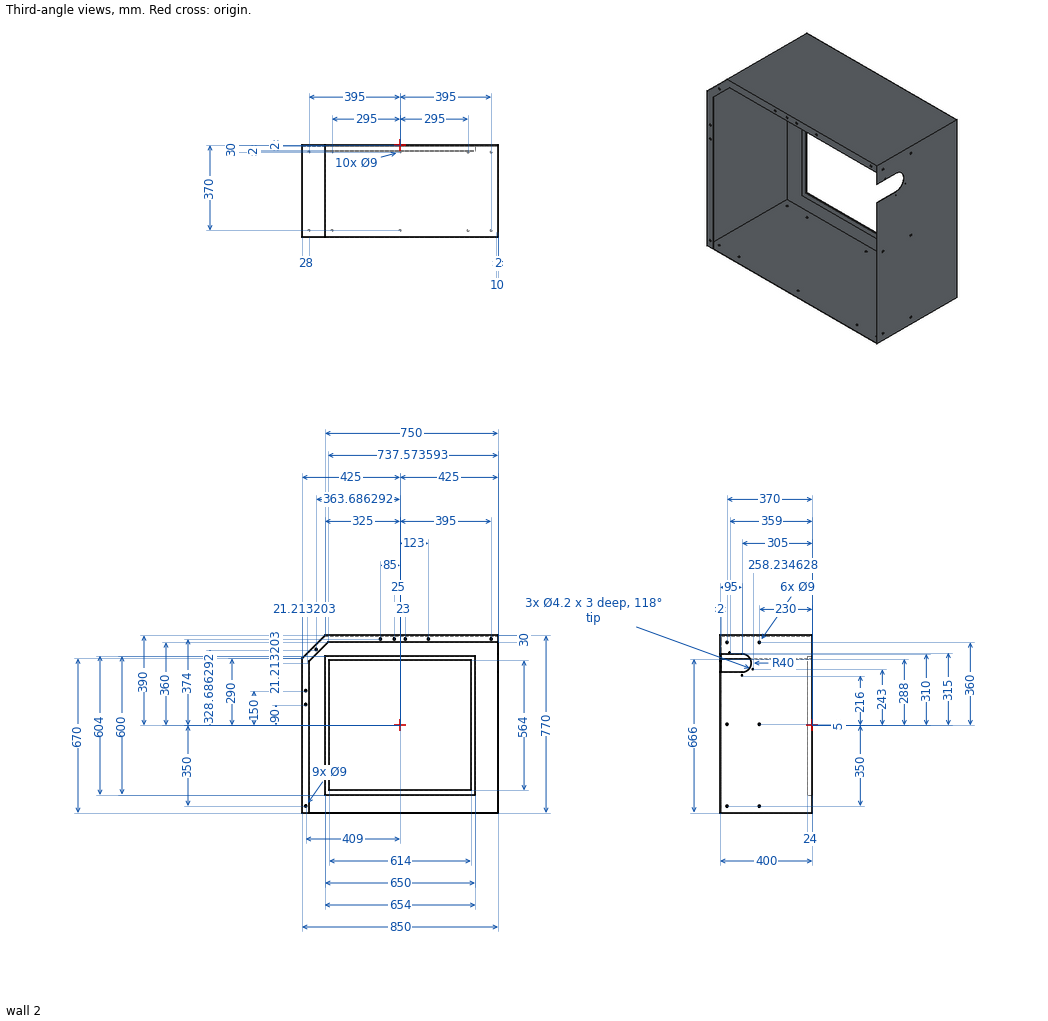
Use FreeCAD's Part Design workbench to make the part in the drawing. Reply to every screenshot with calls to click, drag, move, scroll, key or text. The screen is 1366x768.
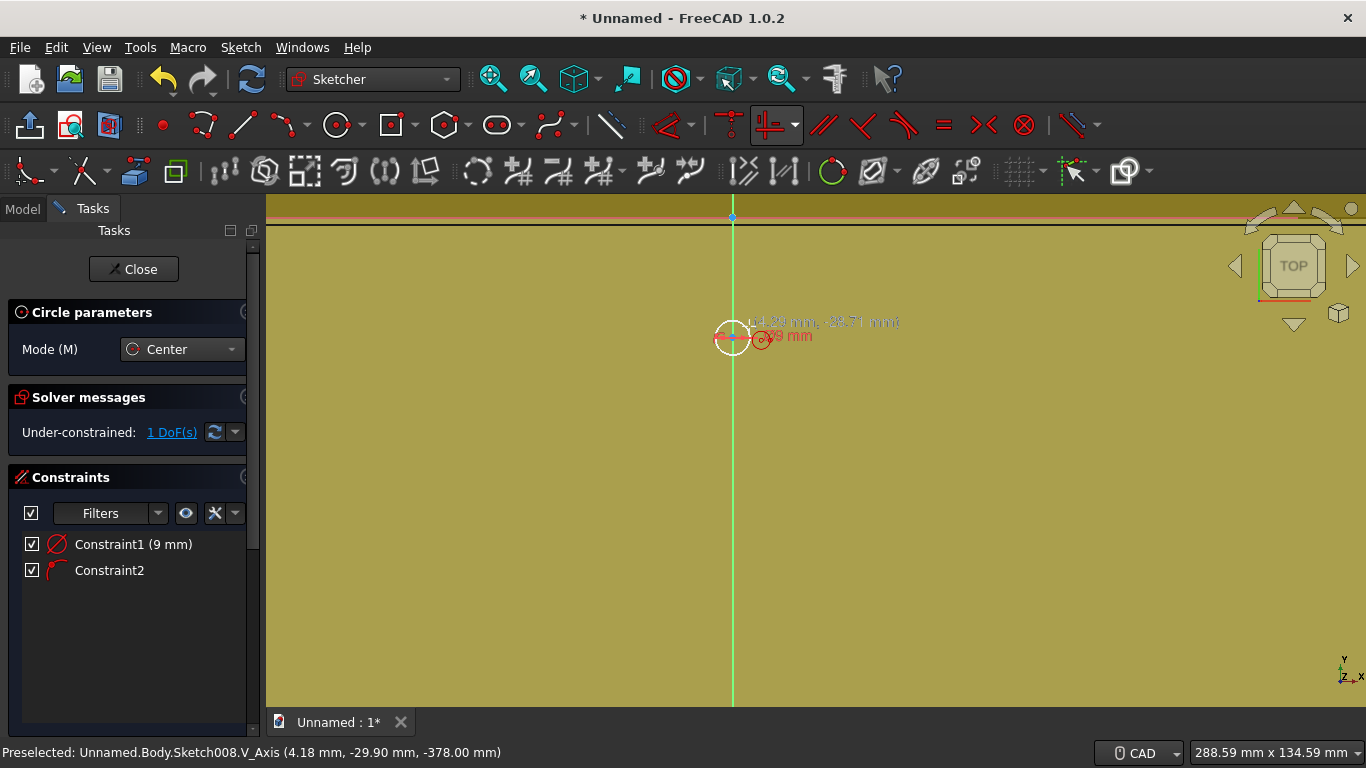
scroll(751, 329, down, 8)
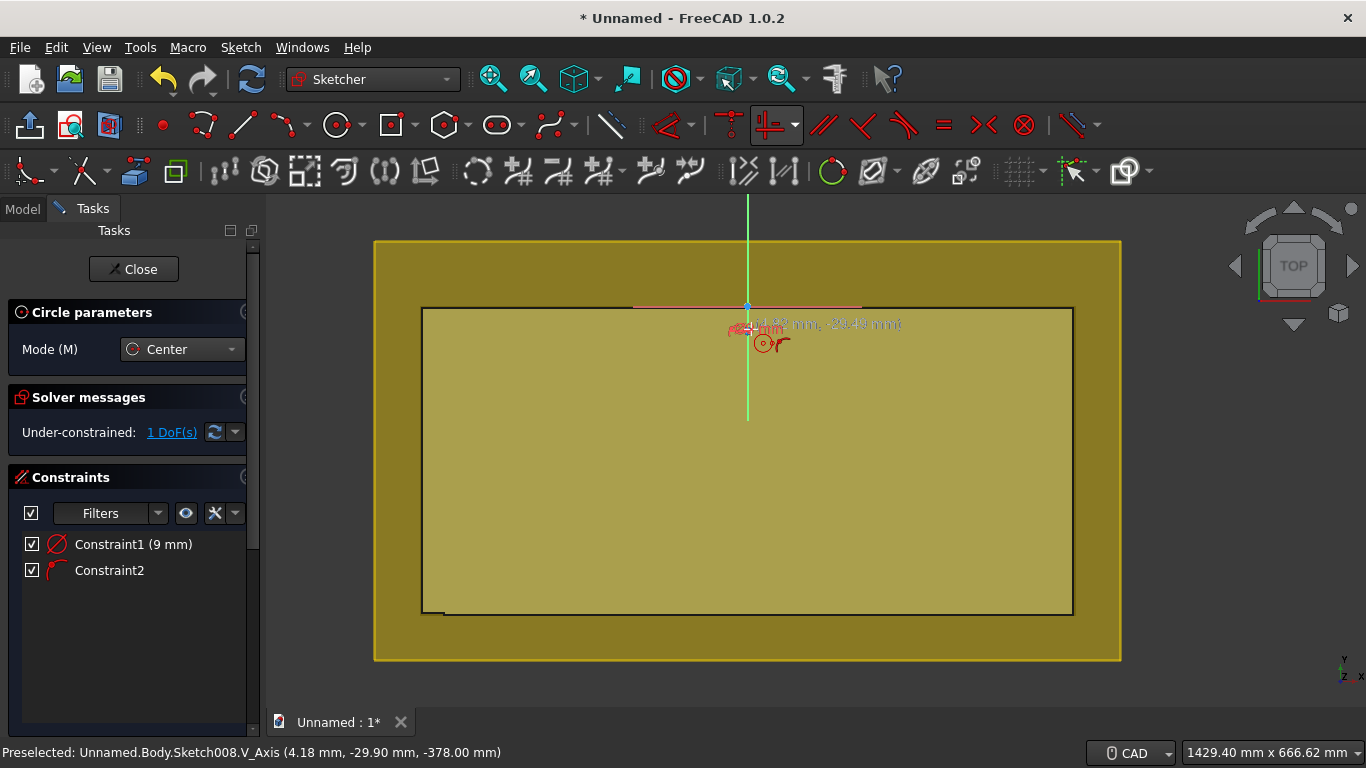
scroll(521, 330, up, 10)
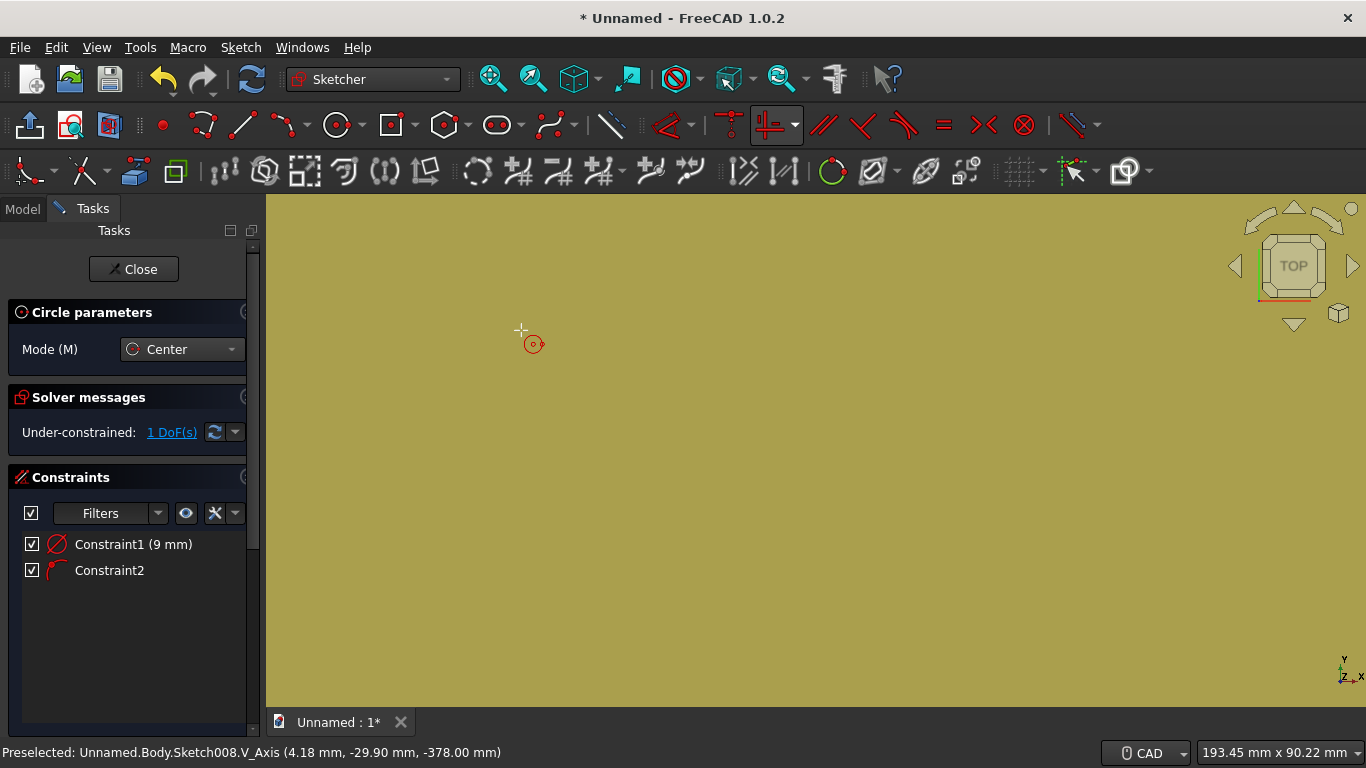
scroll(521, 330, down, 10)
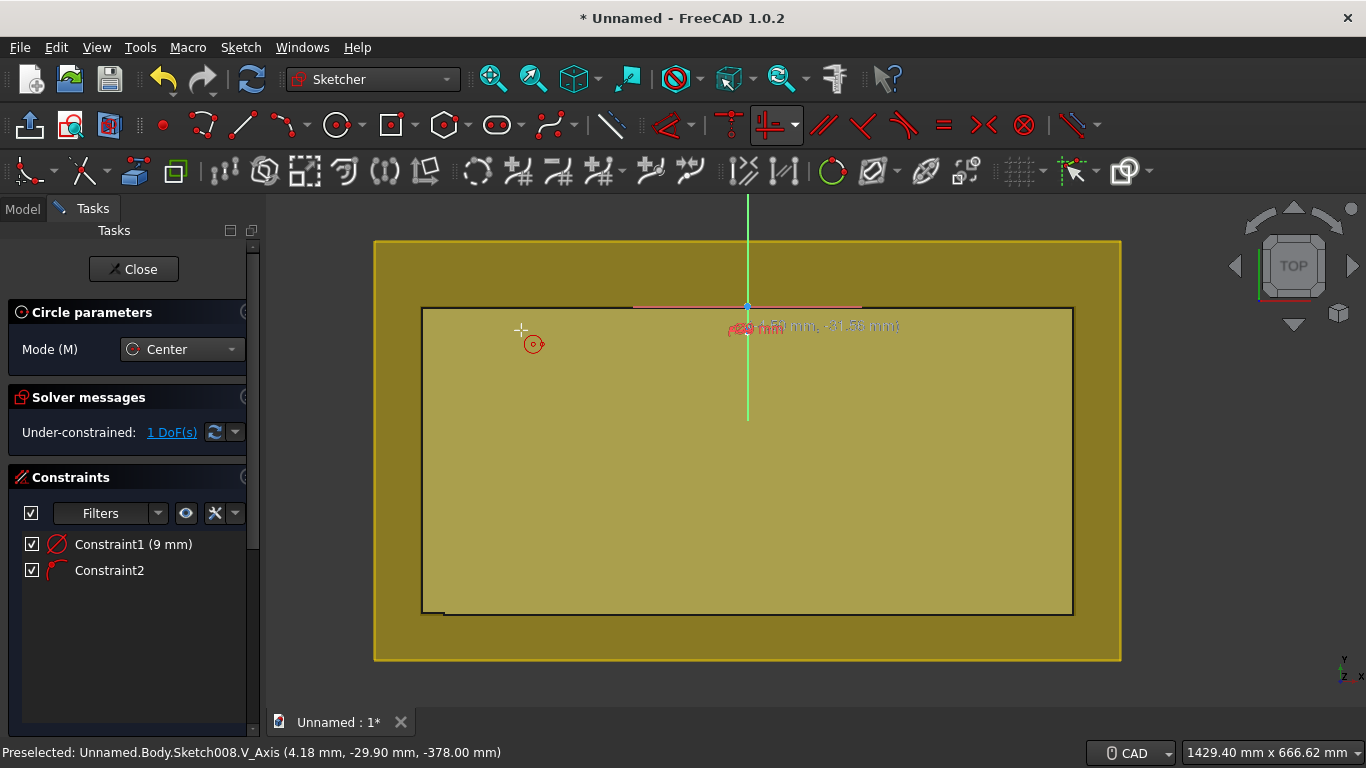
click(521, 330)
move(523, 327)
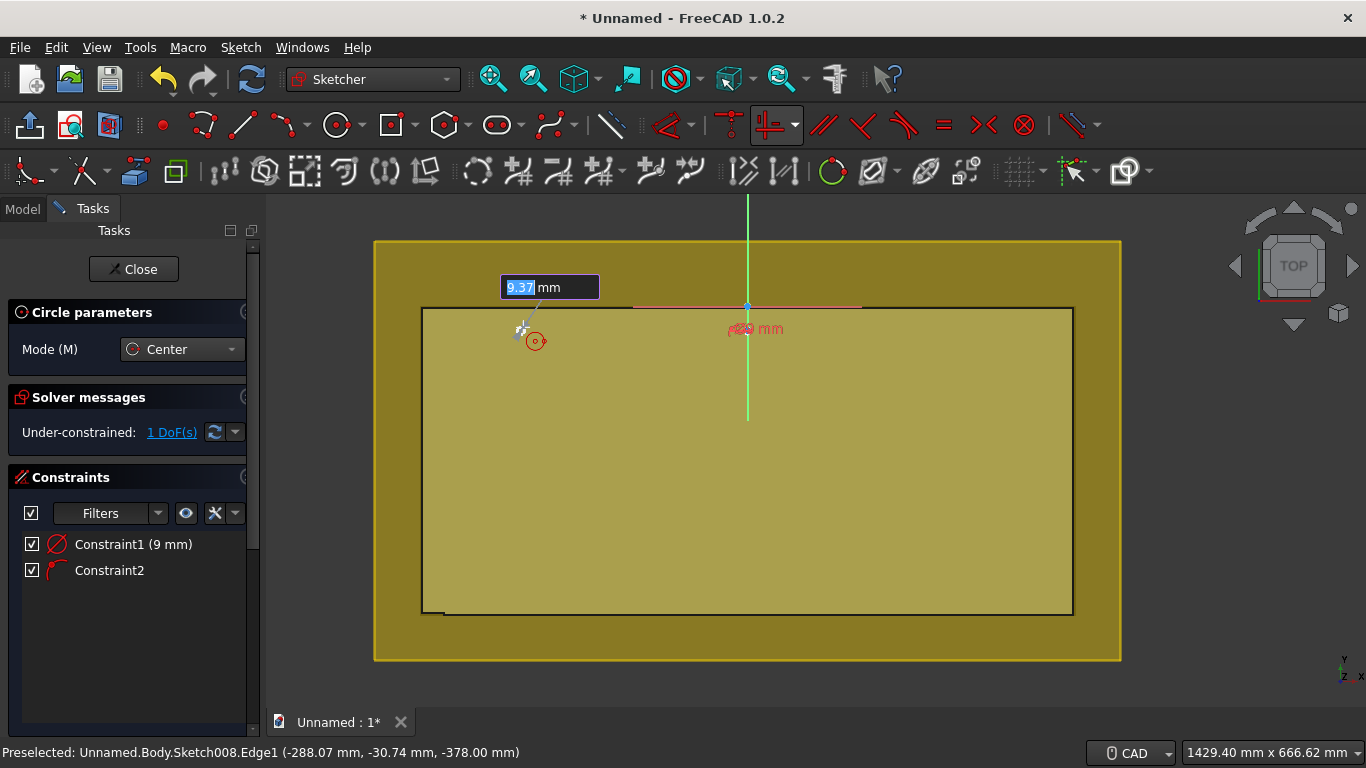
text(9)
key(Return)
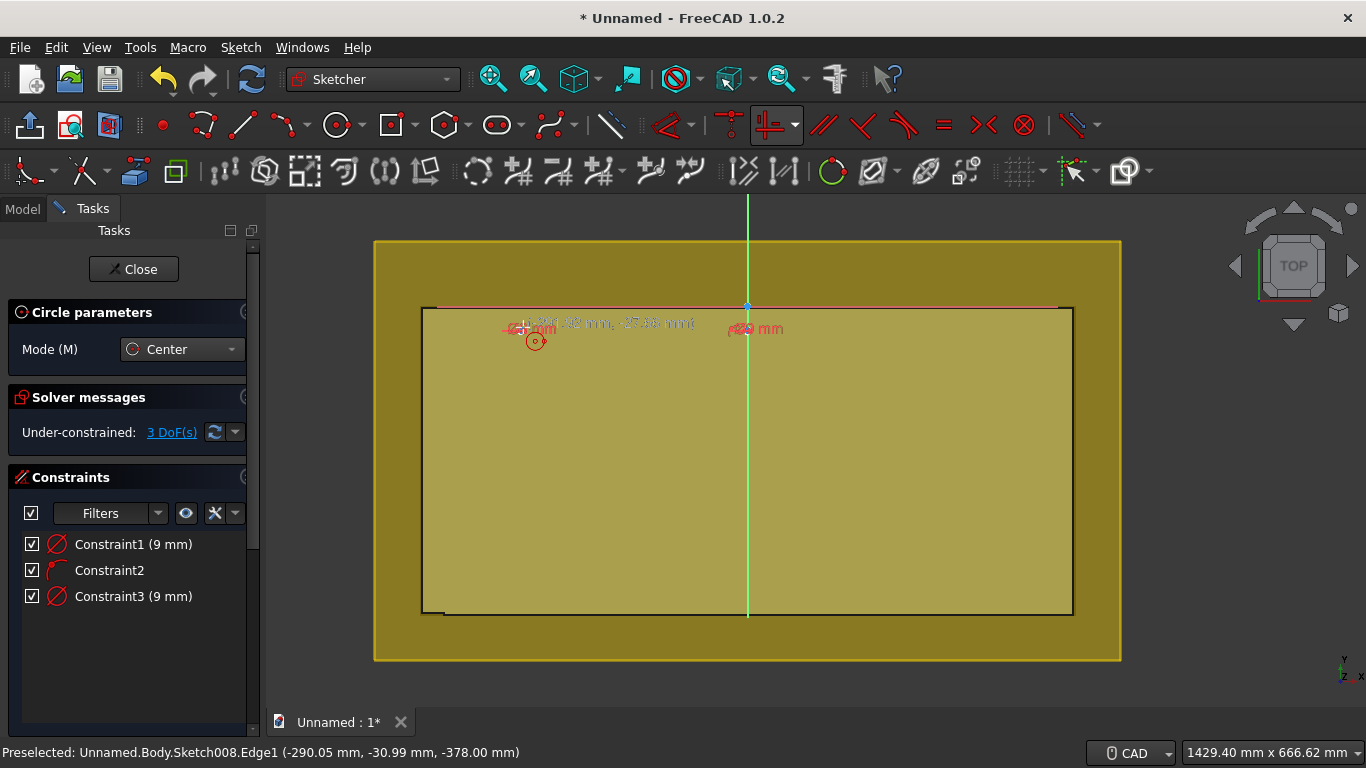
scroll(748, 591, up, 10)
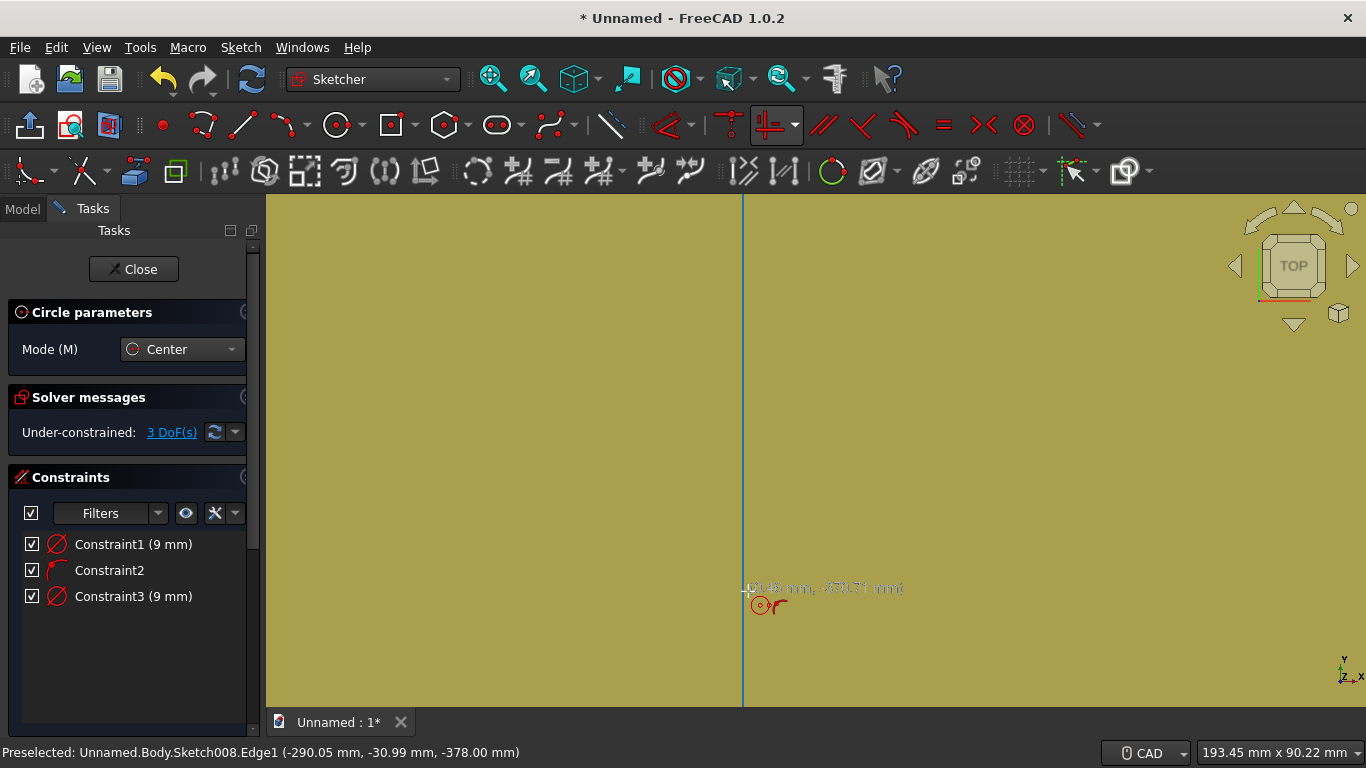
scroll(748, 591, down, 10)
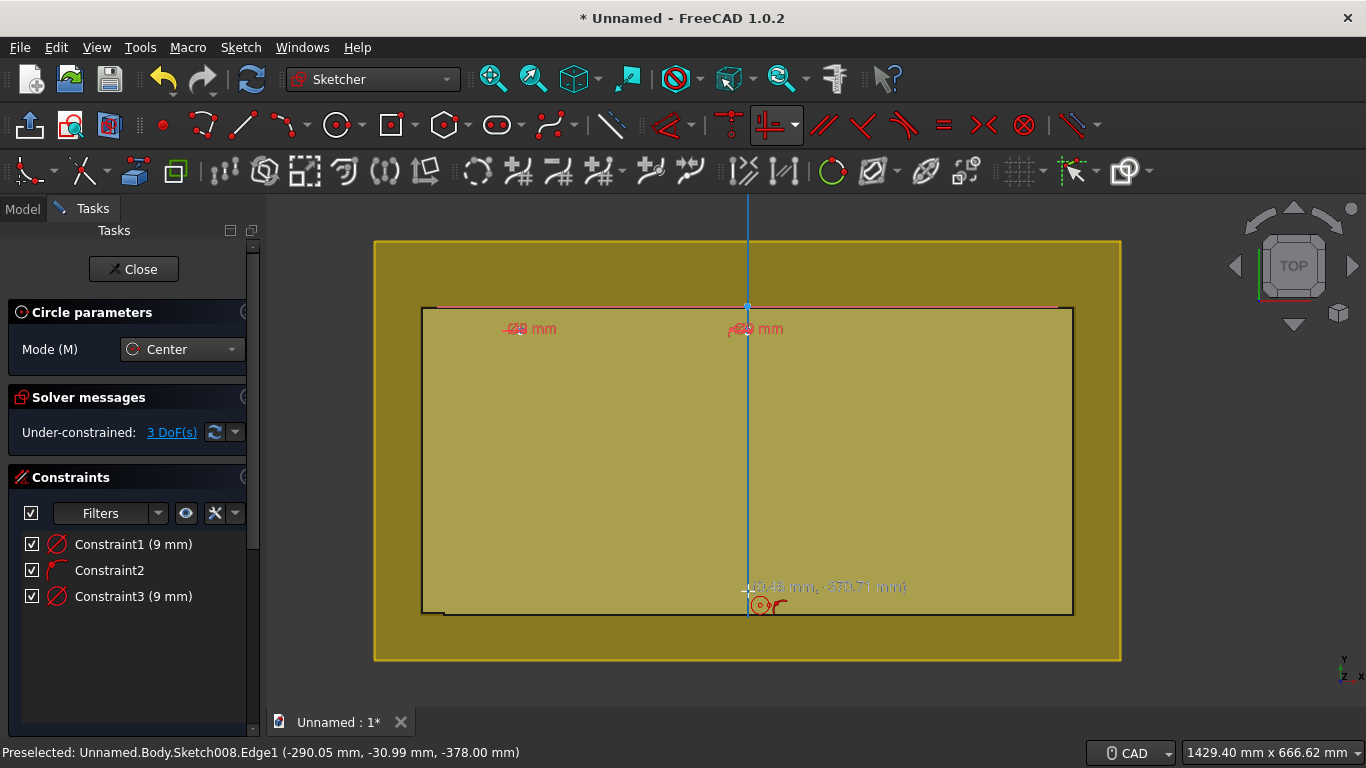
click(748, 591)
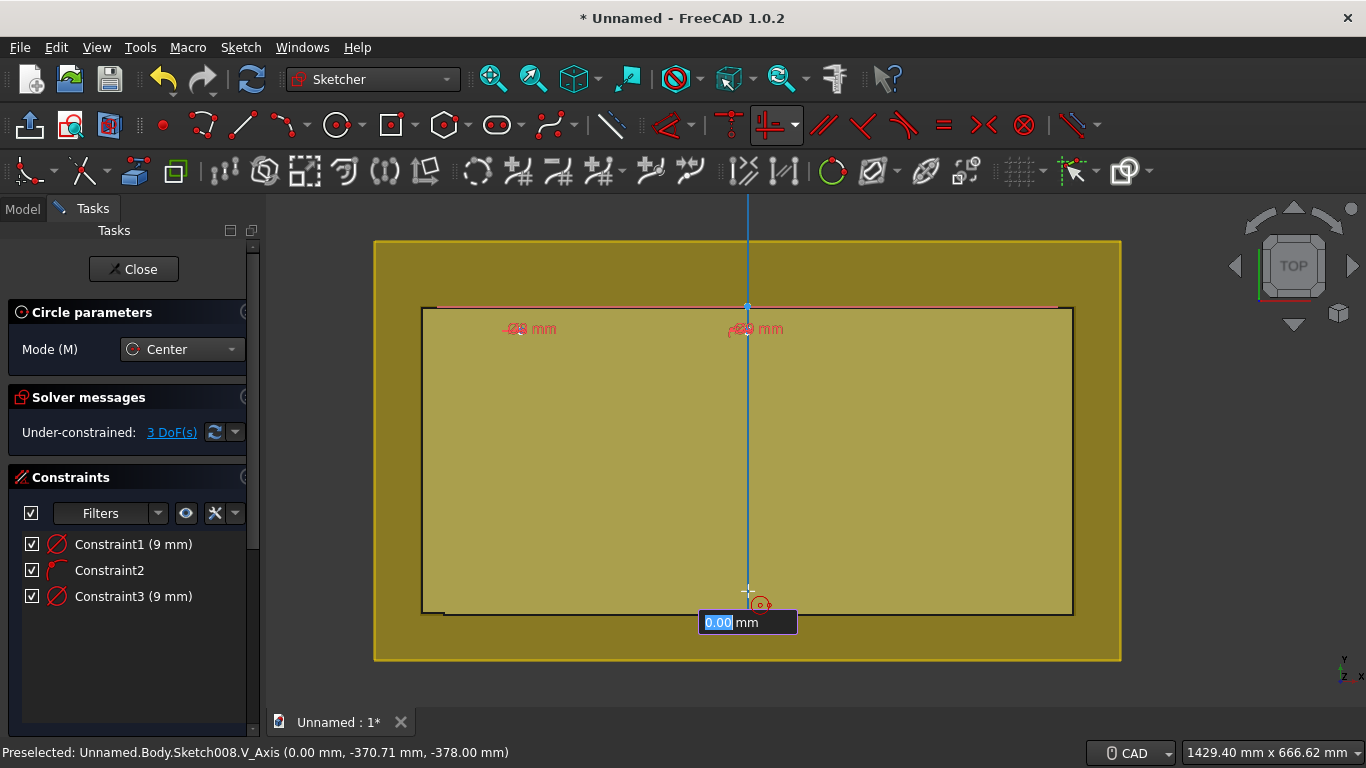
scroll(751, 590, up, 8)
move(749, 588)